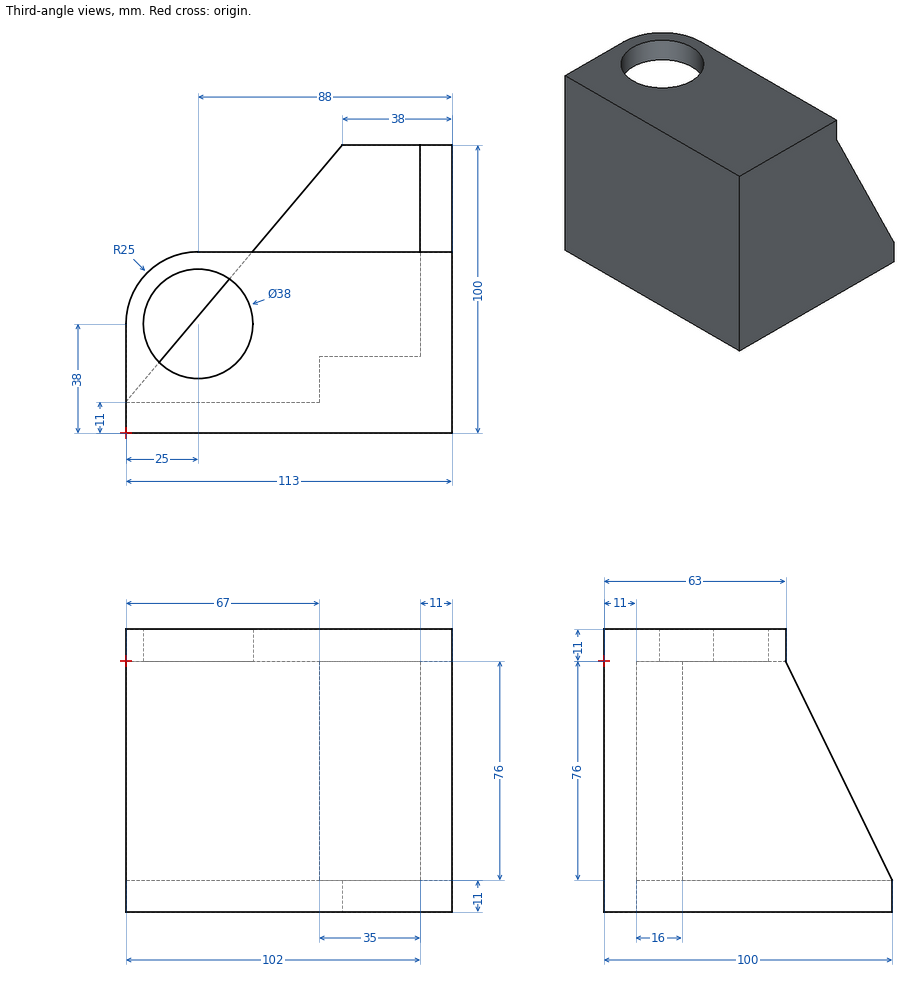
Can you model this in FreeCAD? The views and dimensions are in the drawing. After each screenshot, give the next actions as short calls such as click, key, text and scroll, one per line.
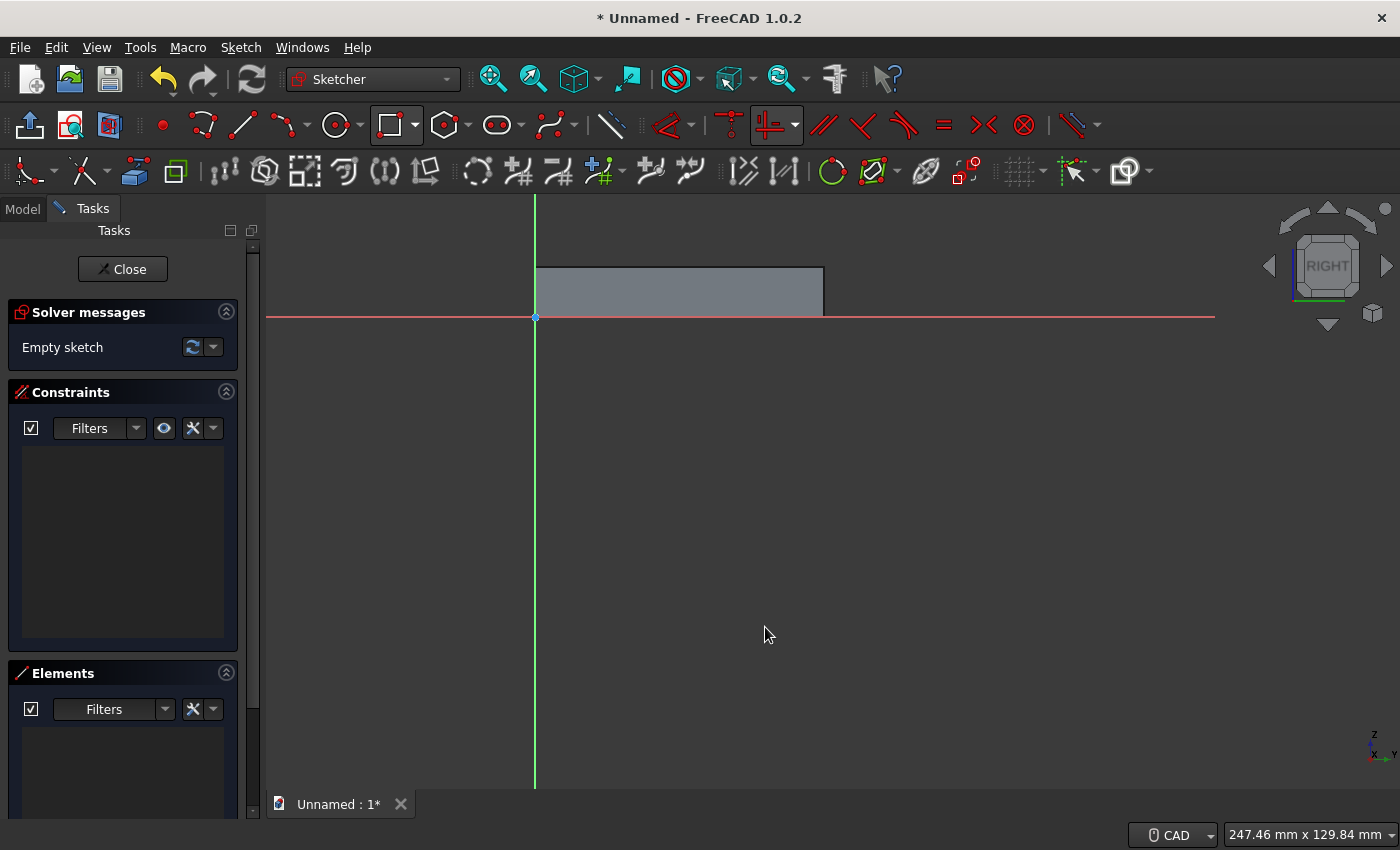
key(g)
key(m)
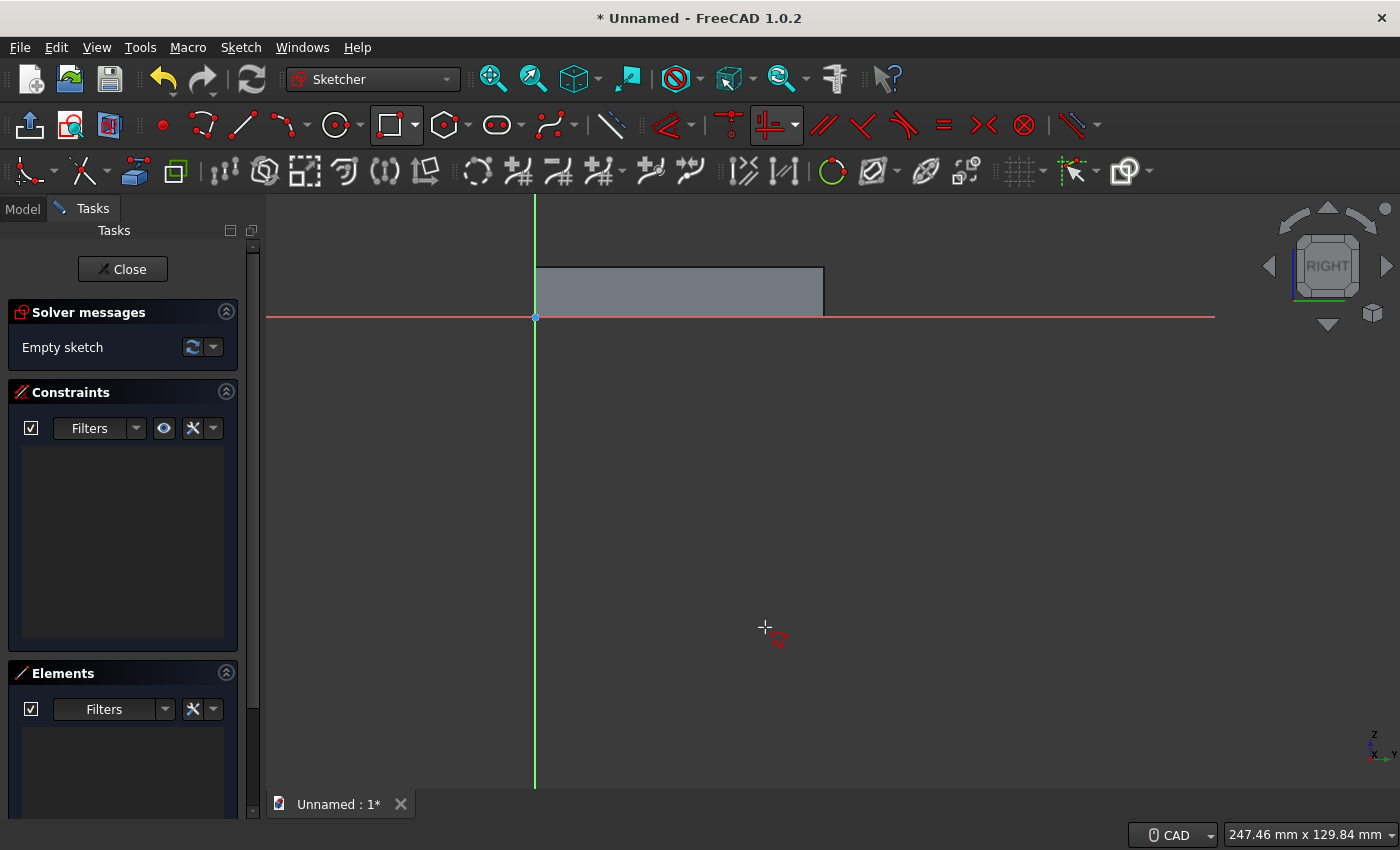
click(535, 317)
click(544, 665)
click(993, 665)
click(824, 326)
click(535, 317)
key(Escape)
key(Escape)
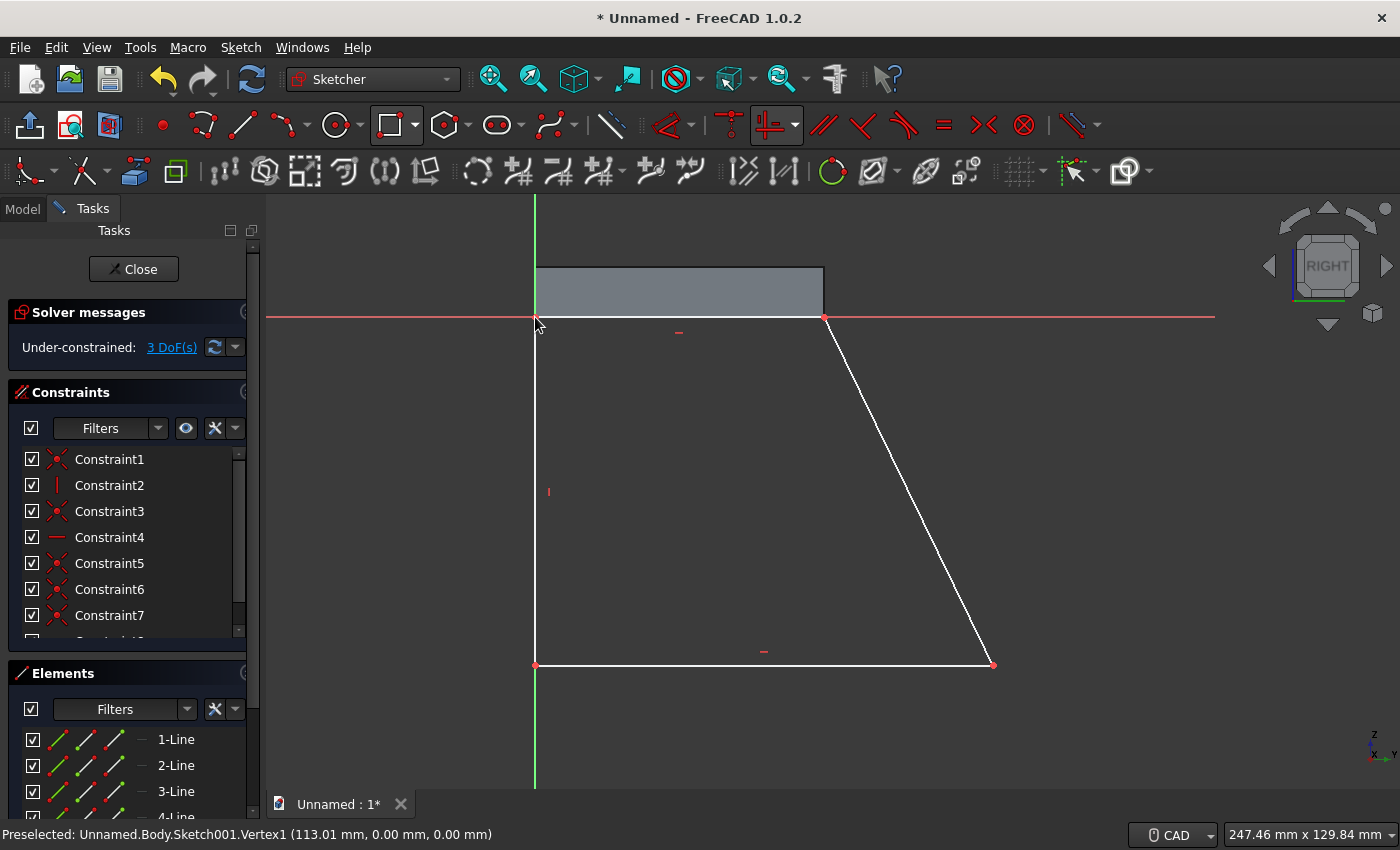
click(666, 126)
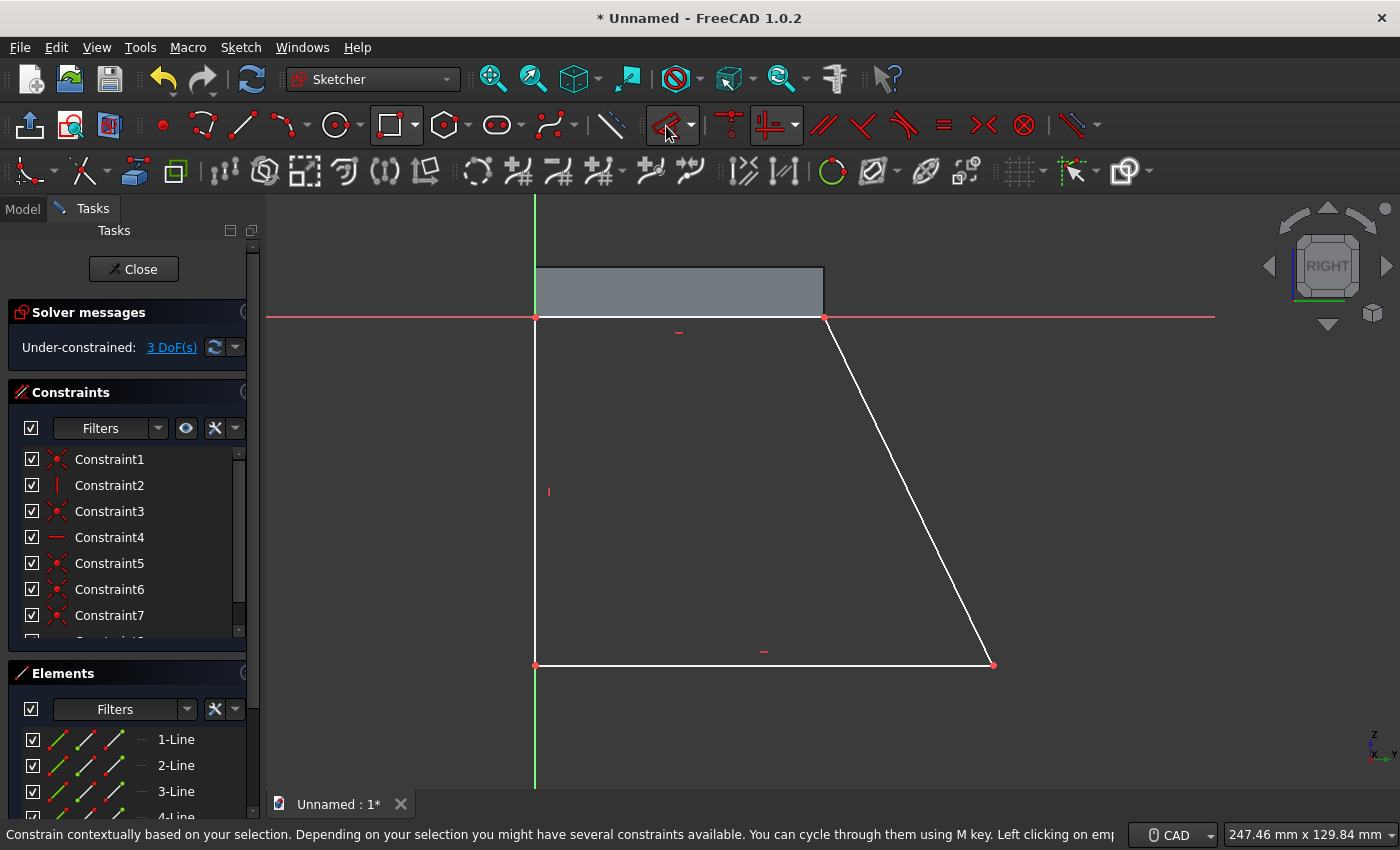
click(535, 422)
click(501, 492)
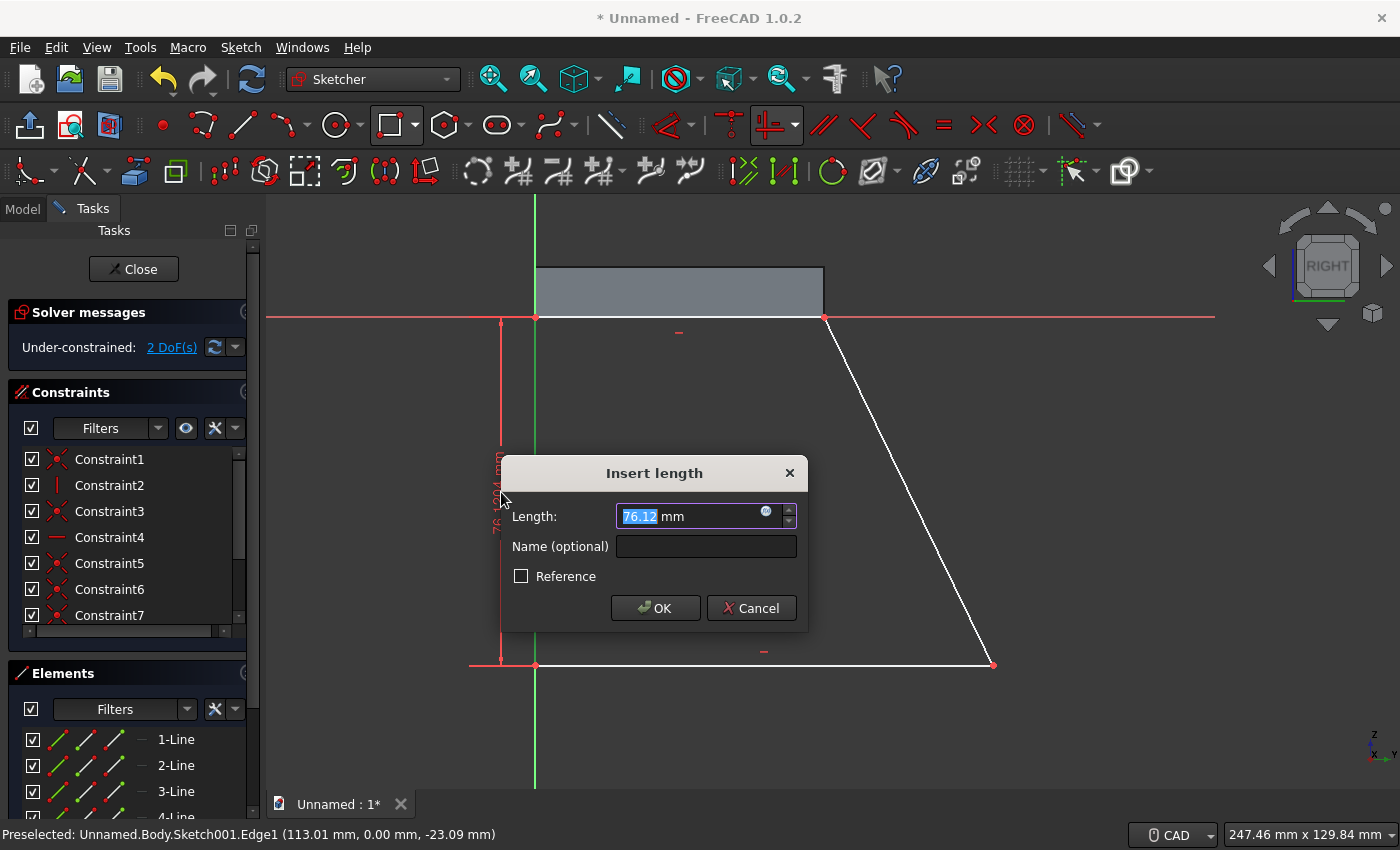
text(76)
key(Return)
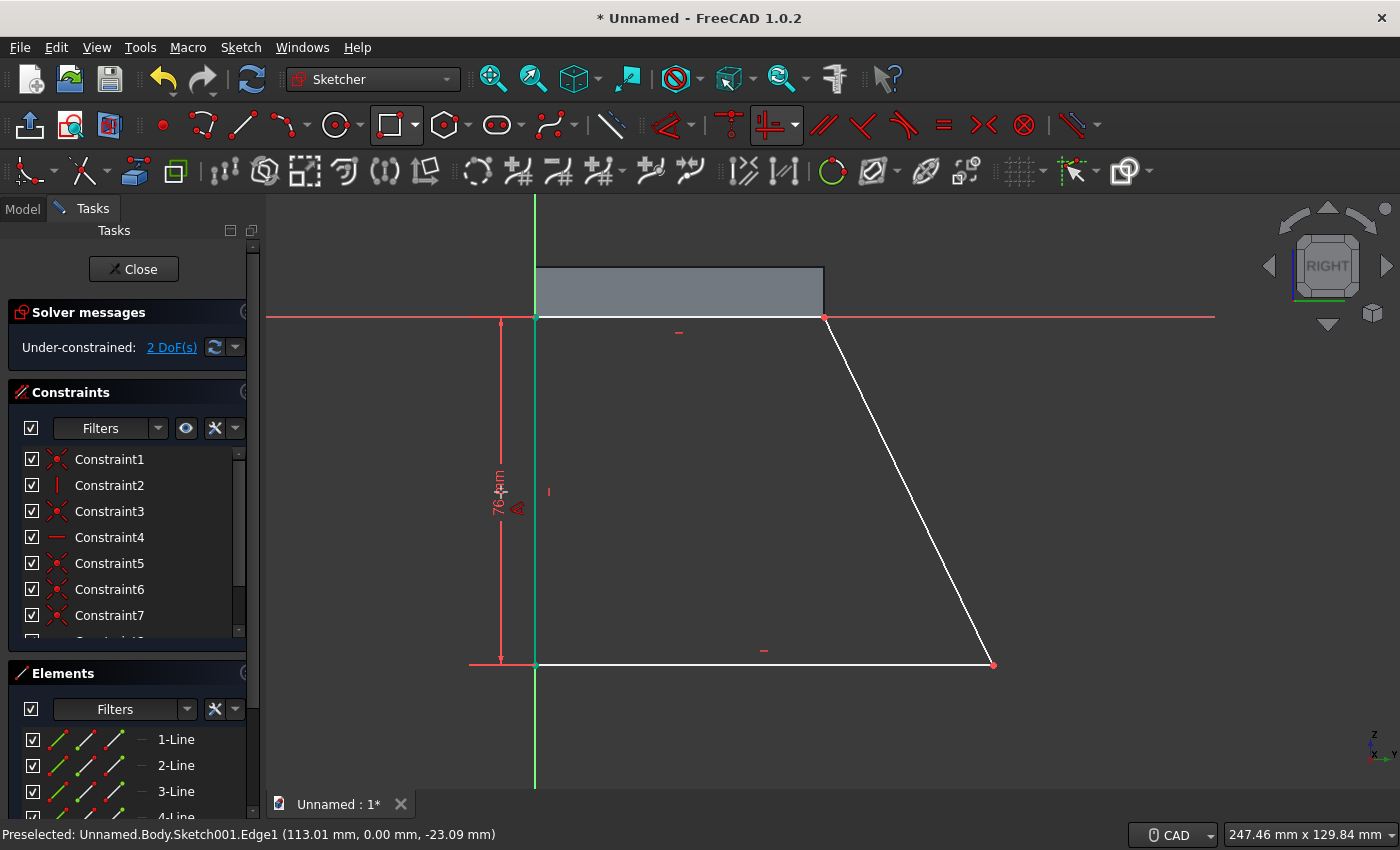
click(737, 317)
click(680, 283)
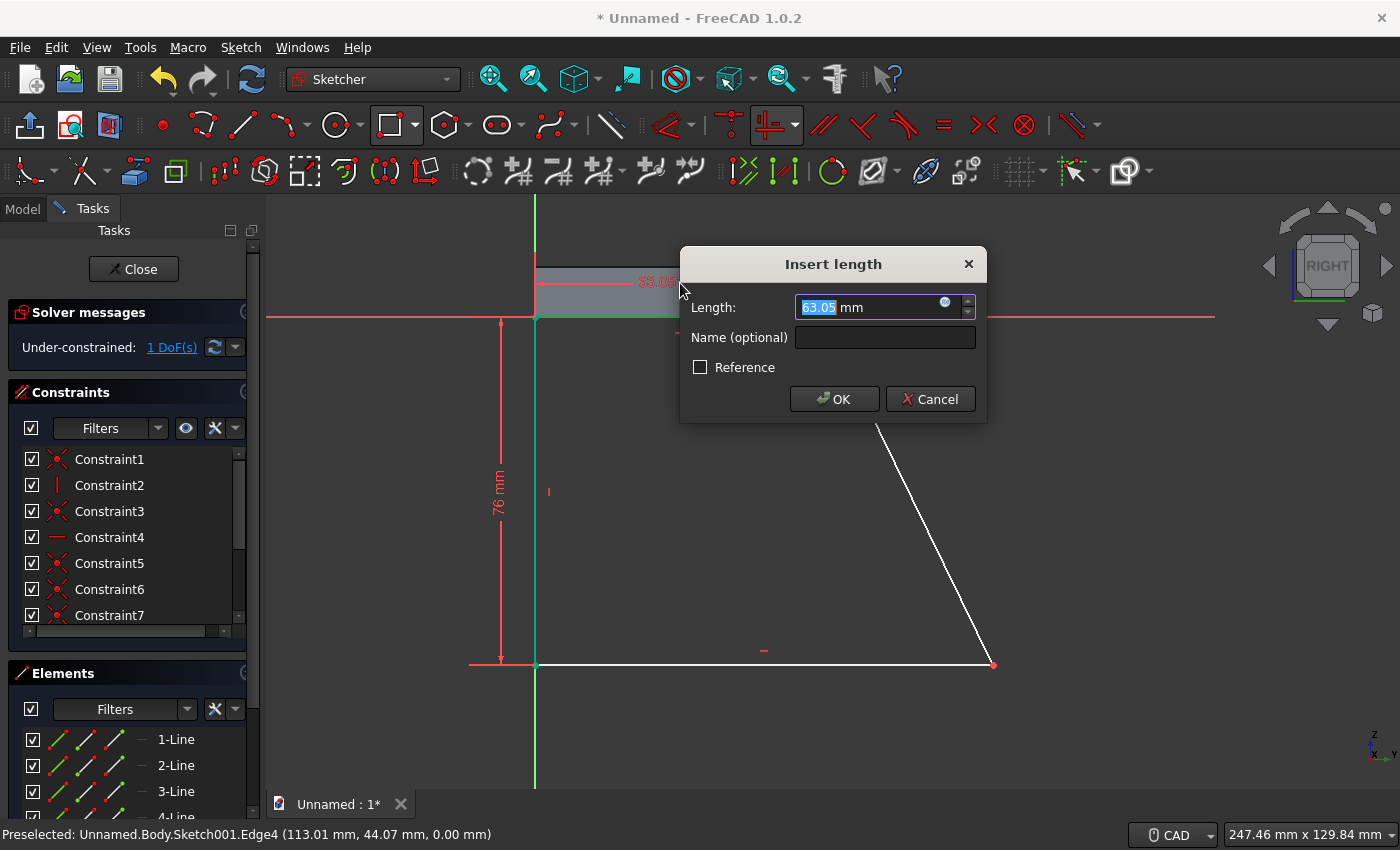
text(63)
key(Return)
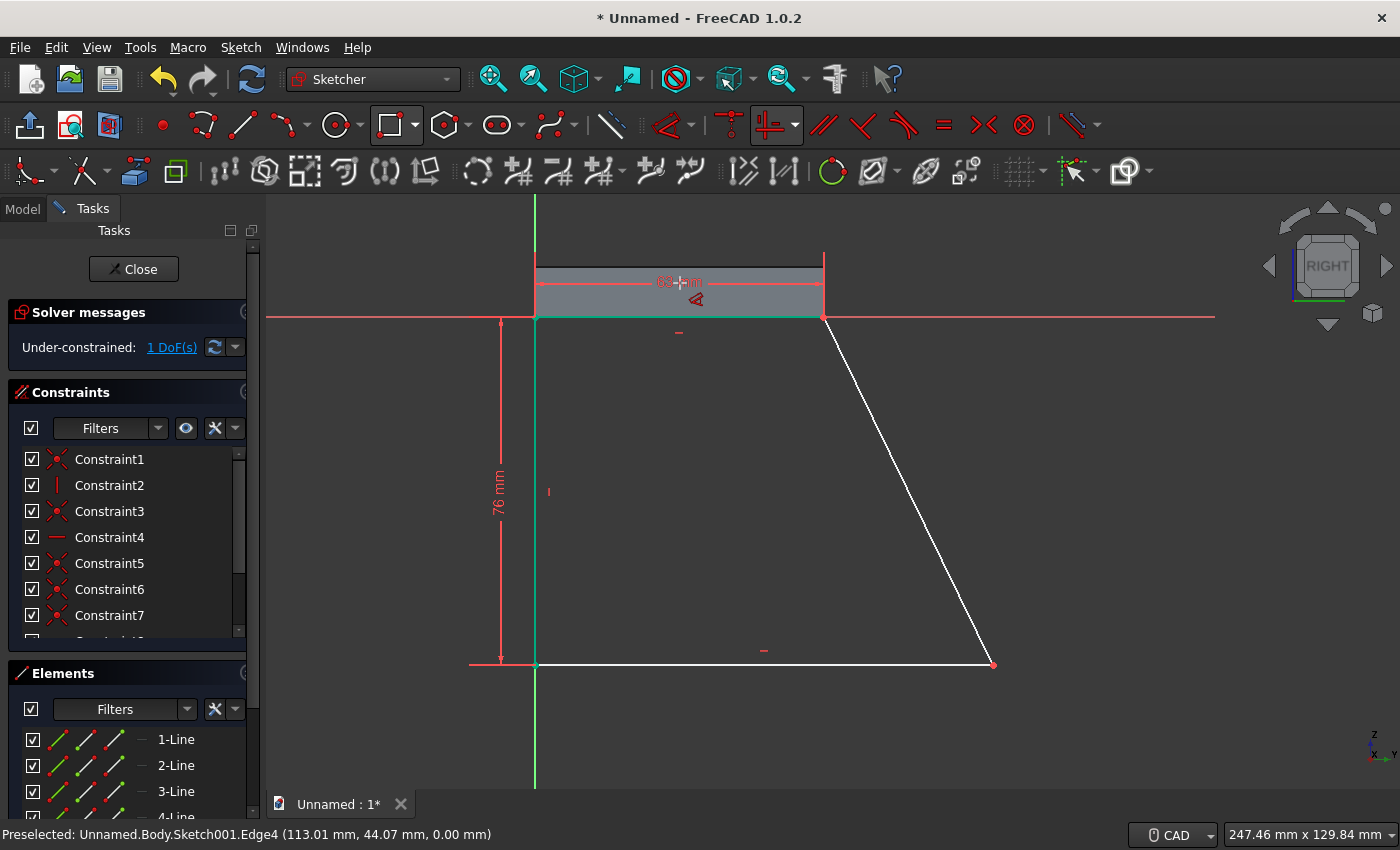
click(672, 665)
click(764, 699)